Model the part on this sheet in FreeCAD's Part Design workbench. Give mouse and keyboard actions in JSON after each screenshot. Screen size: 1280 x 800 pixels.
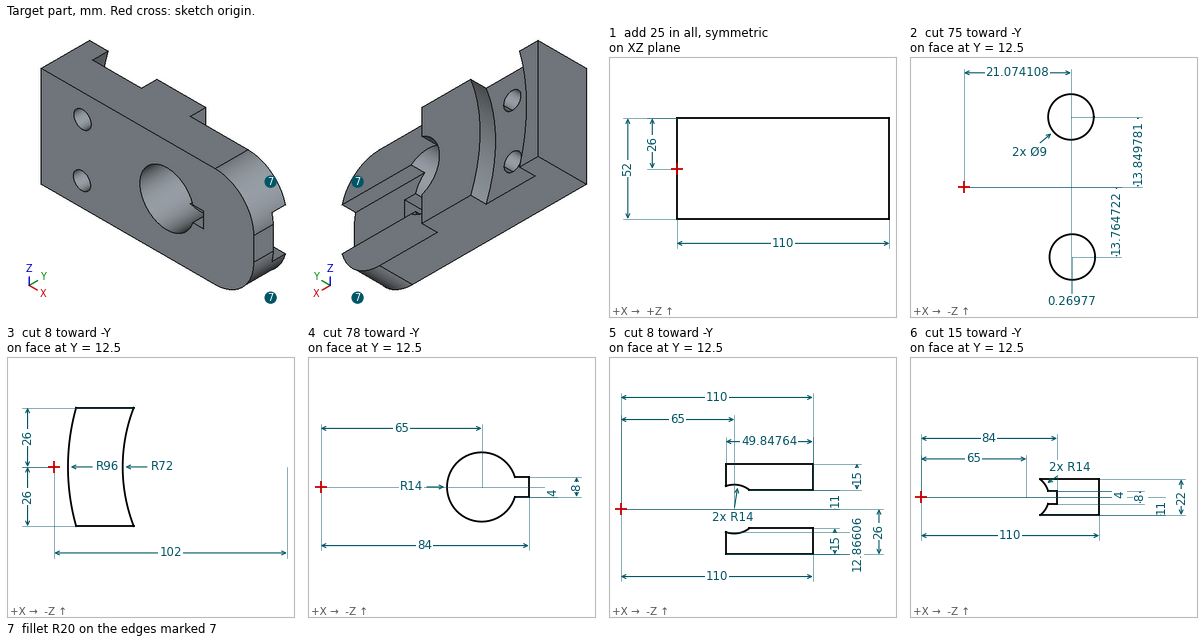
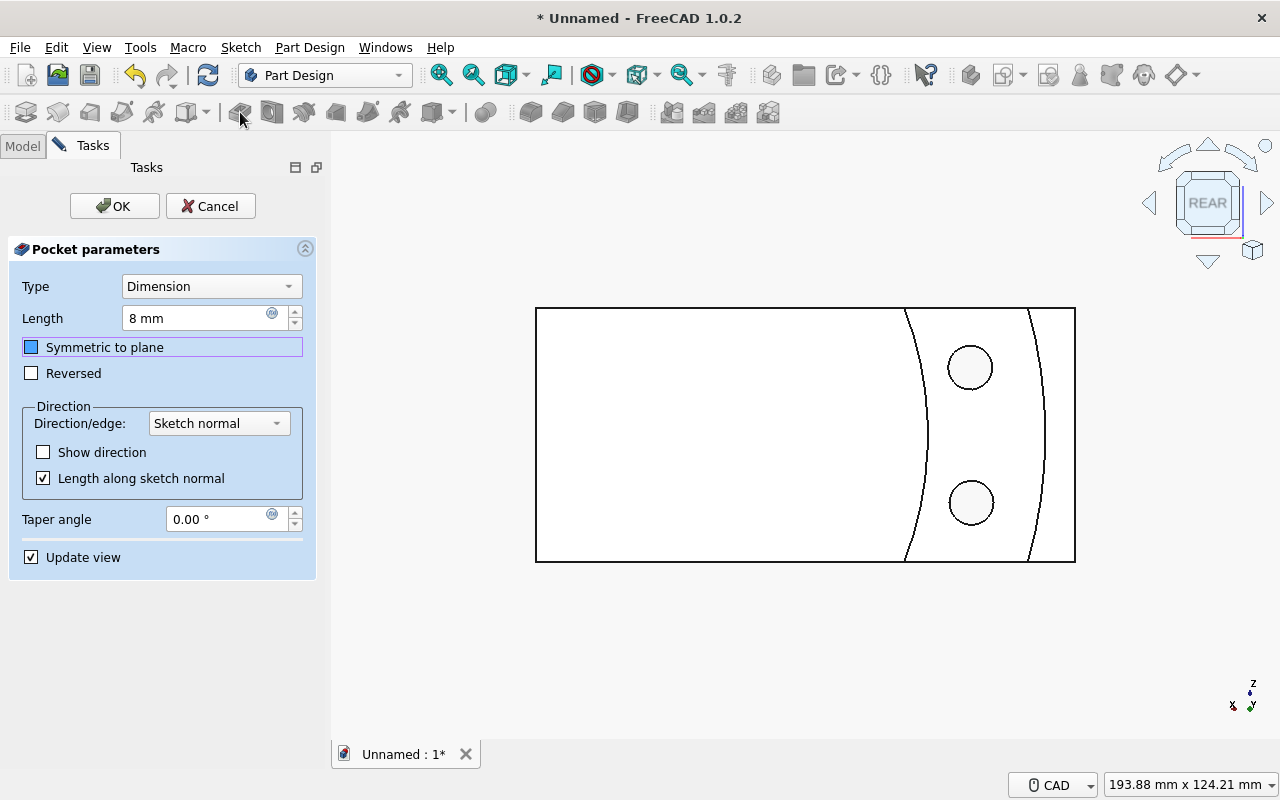
{"action": "left_click", "coordinate": [115, 206]}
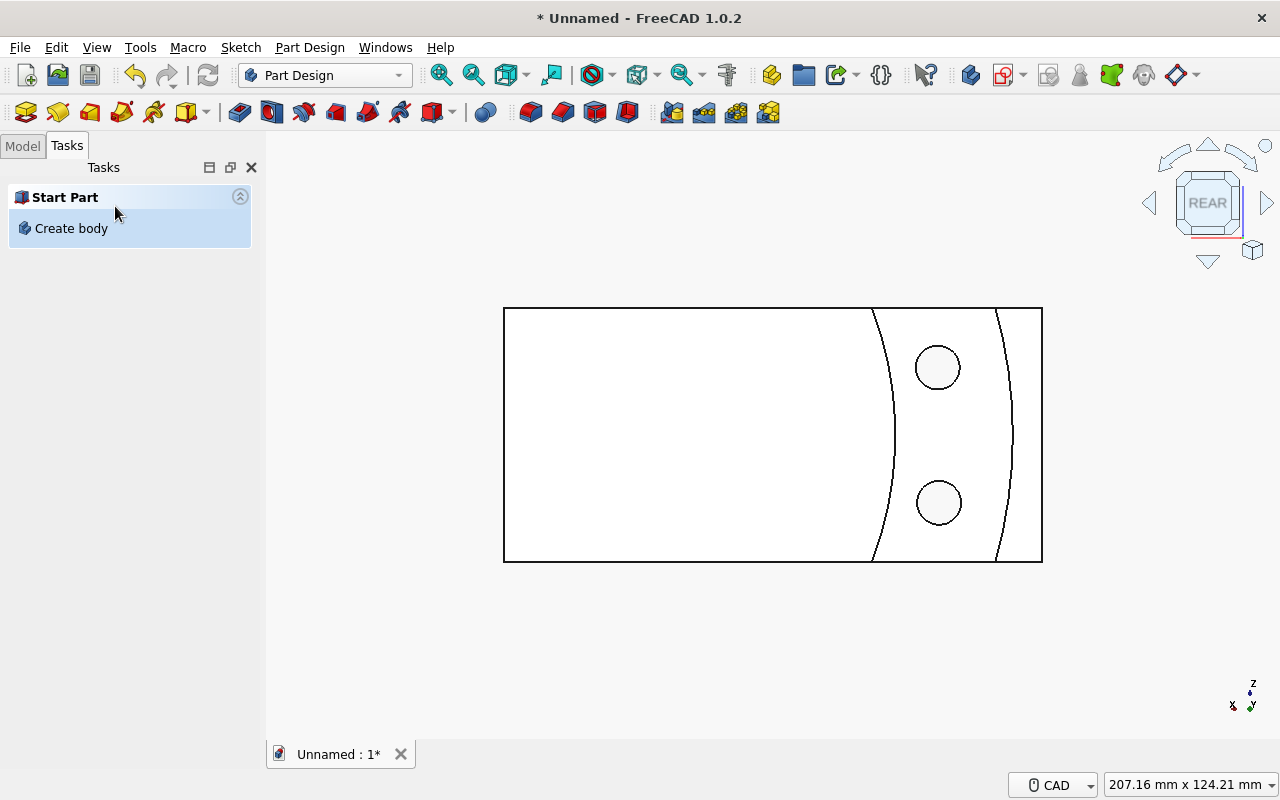
{"action": "left_click", "coordinate": [644, 434]}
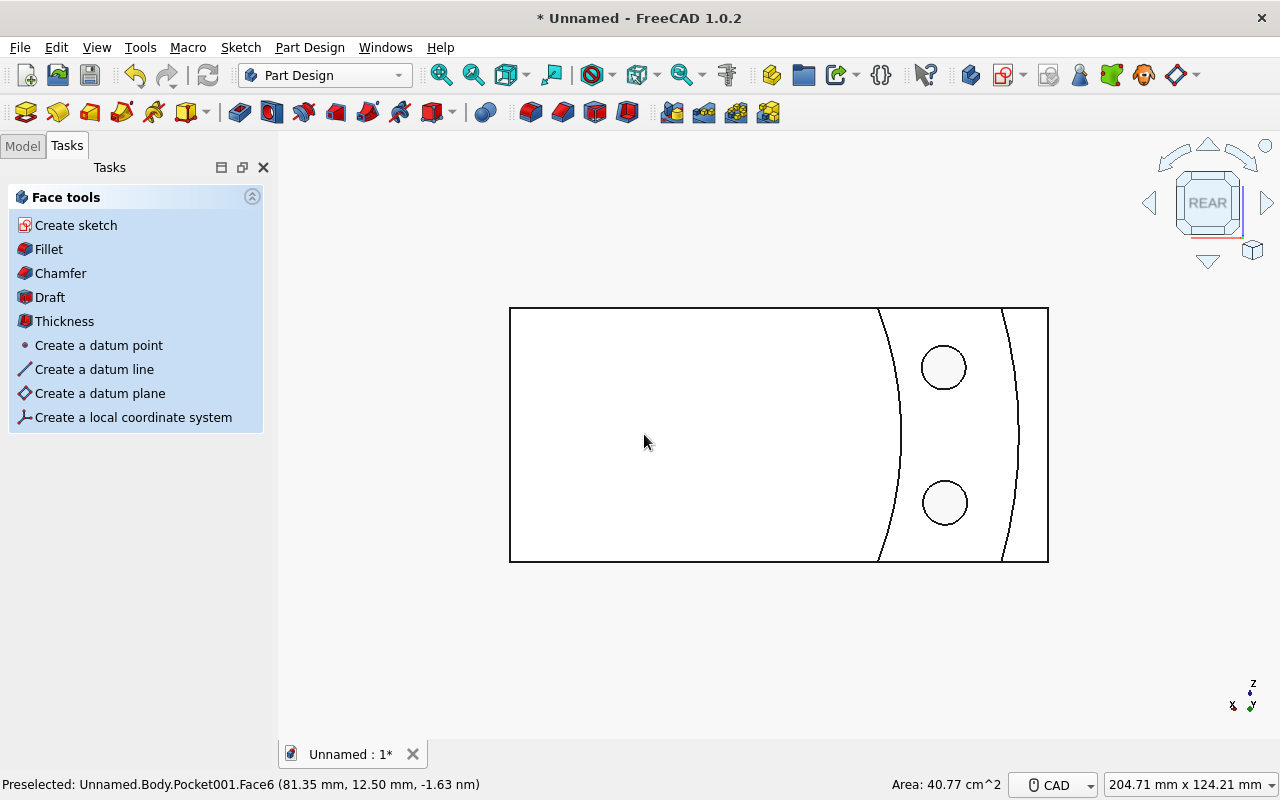
{"action": "left_click", "coordinate": [1004, 76]}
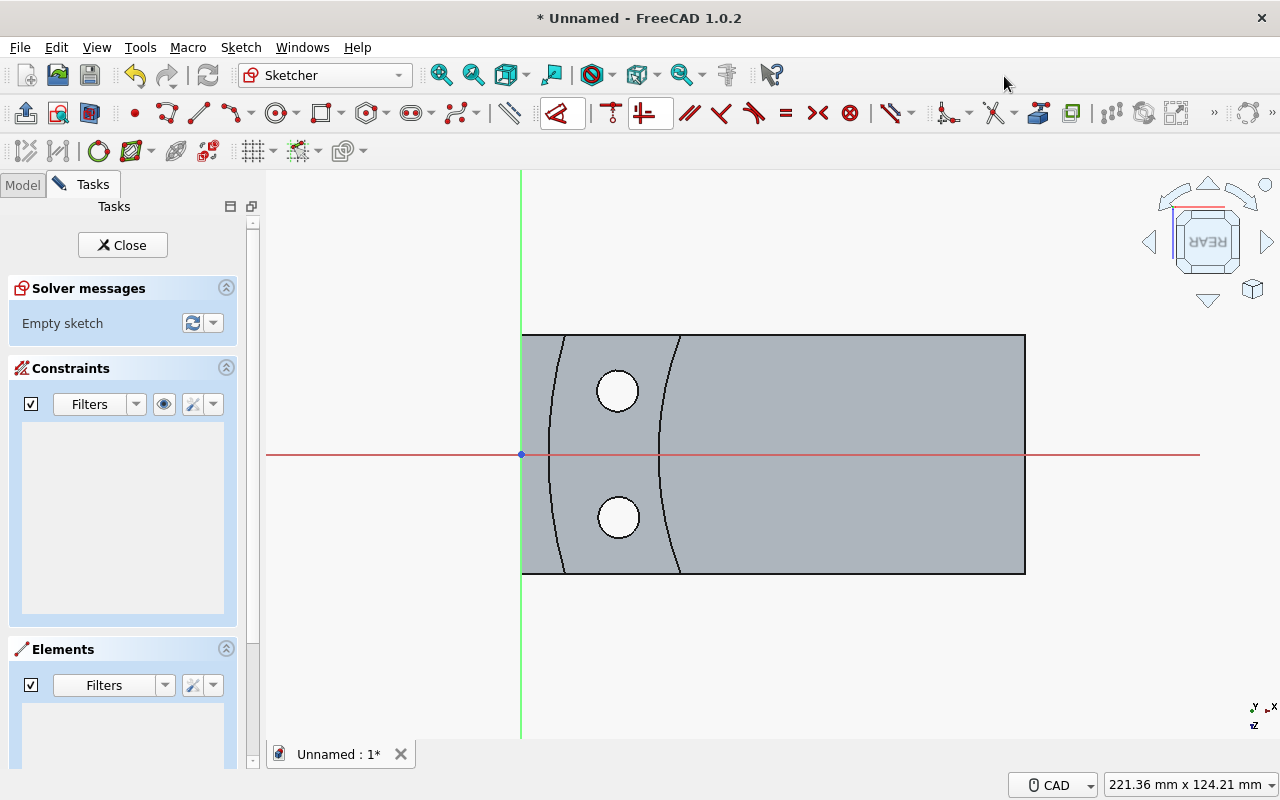
{"action": "scroll", "coordinate": [871, 454], "scroll_direction": "up", "scroll_amount": 7}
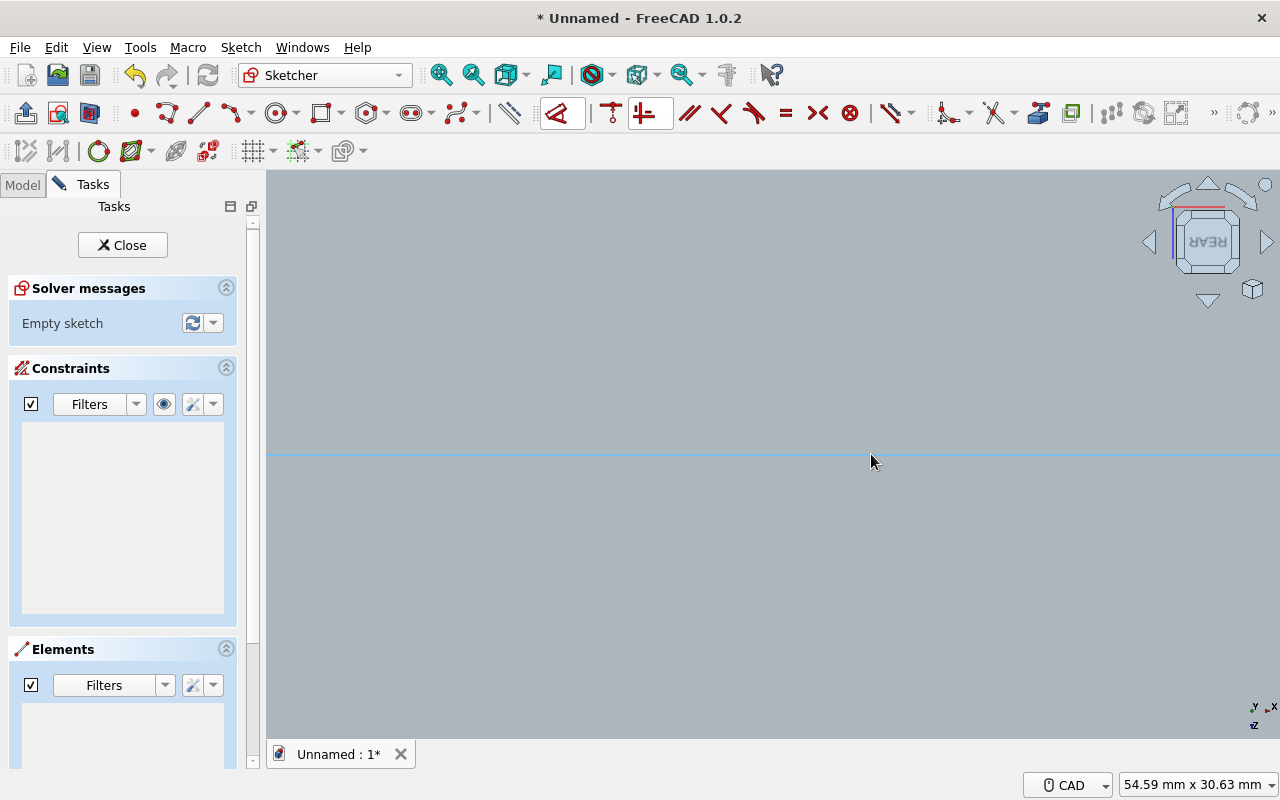
{"action": "left_click", "coordinate": [168, 114]}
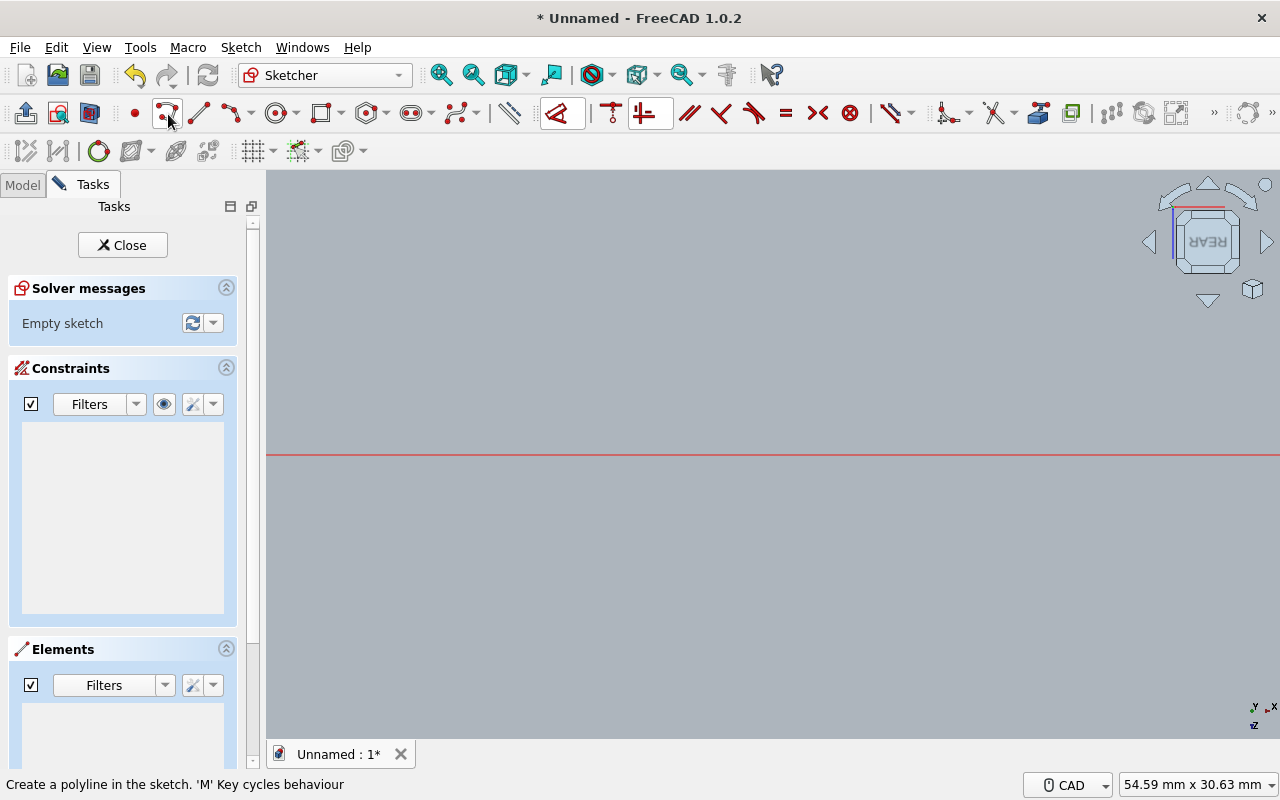
{"action": "left_click", "coordinate": [907, 529]}
{"action": "left_click", "coordinate": [1010, 529]}
{"action": "left_click", "coordinate": [1010, 380]}
{"action": "left_click", "coordinate": [907, 380]}
{"action": "right_click", "coordinate": [907, 380]}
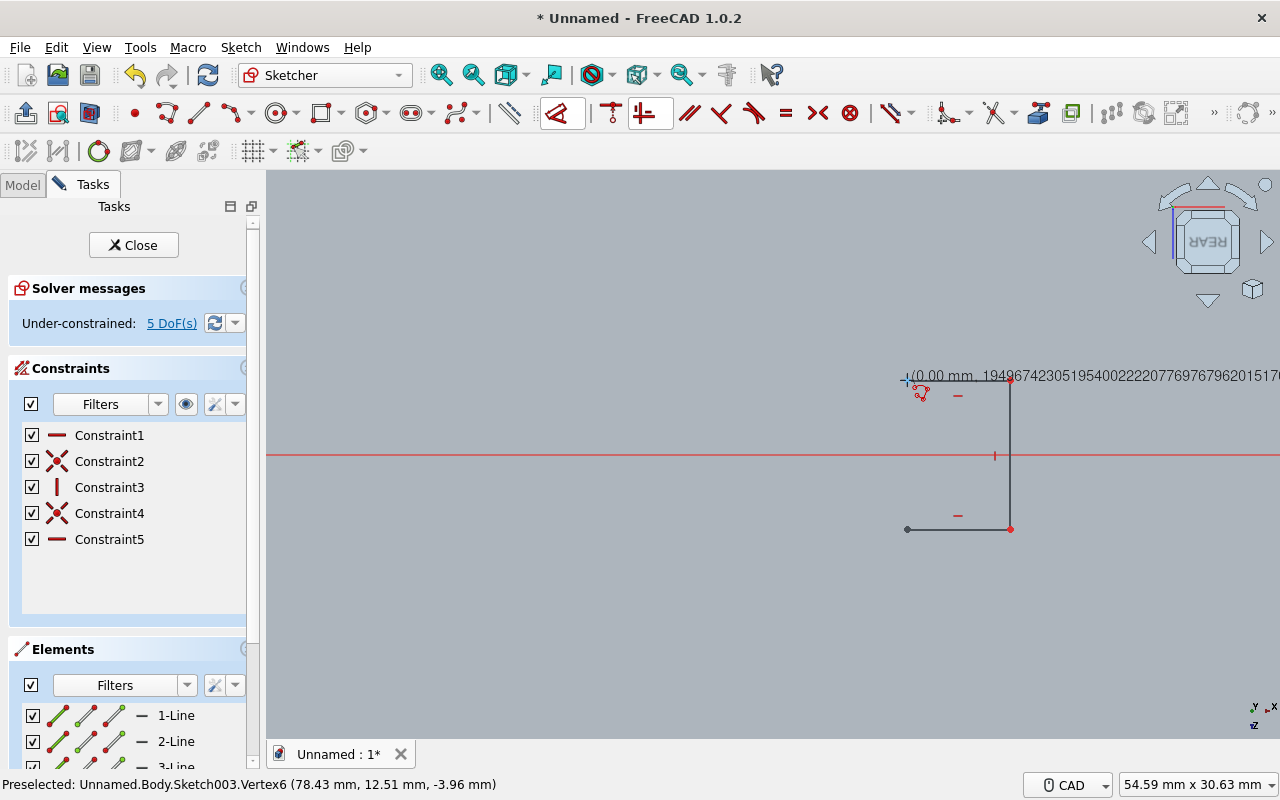
{"action": "left_click", "coordinate": [232, 114]}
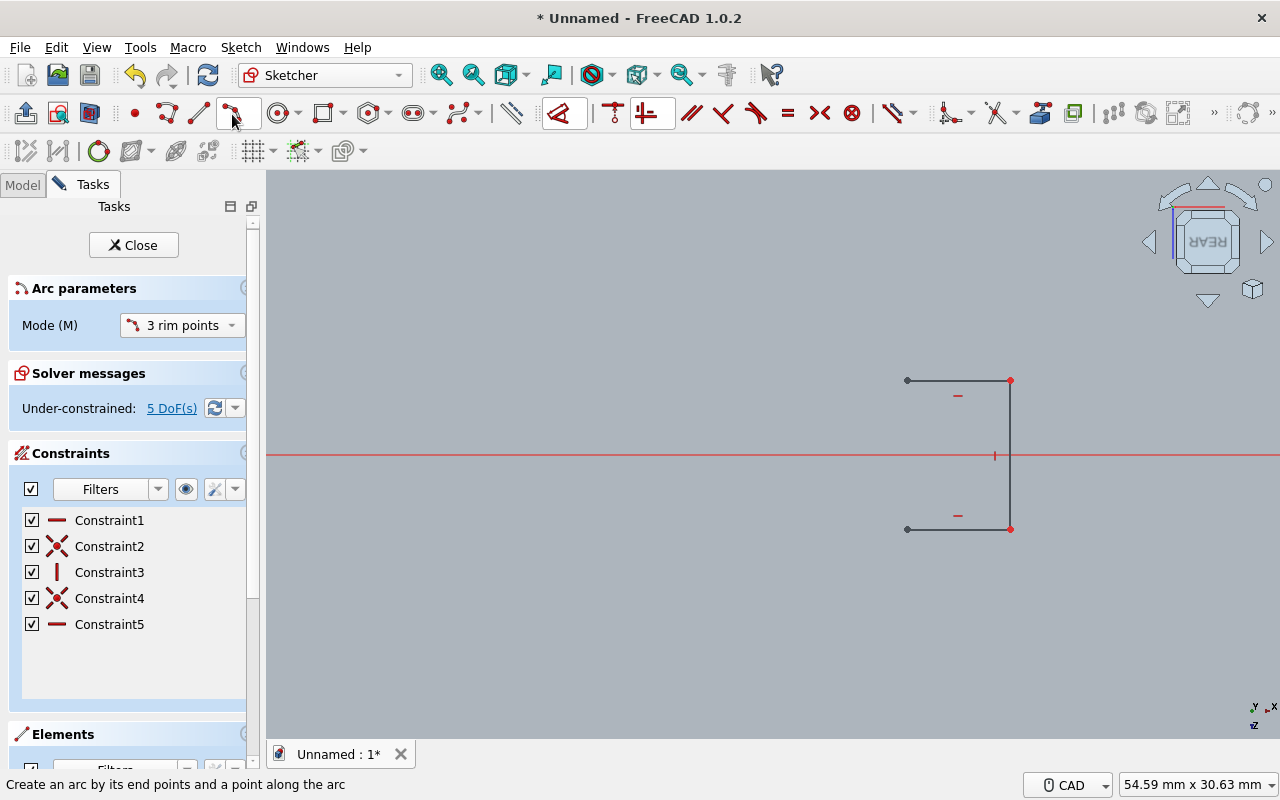
{"action": "left_click", "coordinate": [907, 381]}
{"action": "left_click", "coordinate": [907, 530]}
{"action": "left_click", "coordinate": [439, 314]}
{"action": "key", "text": "Escape"}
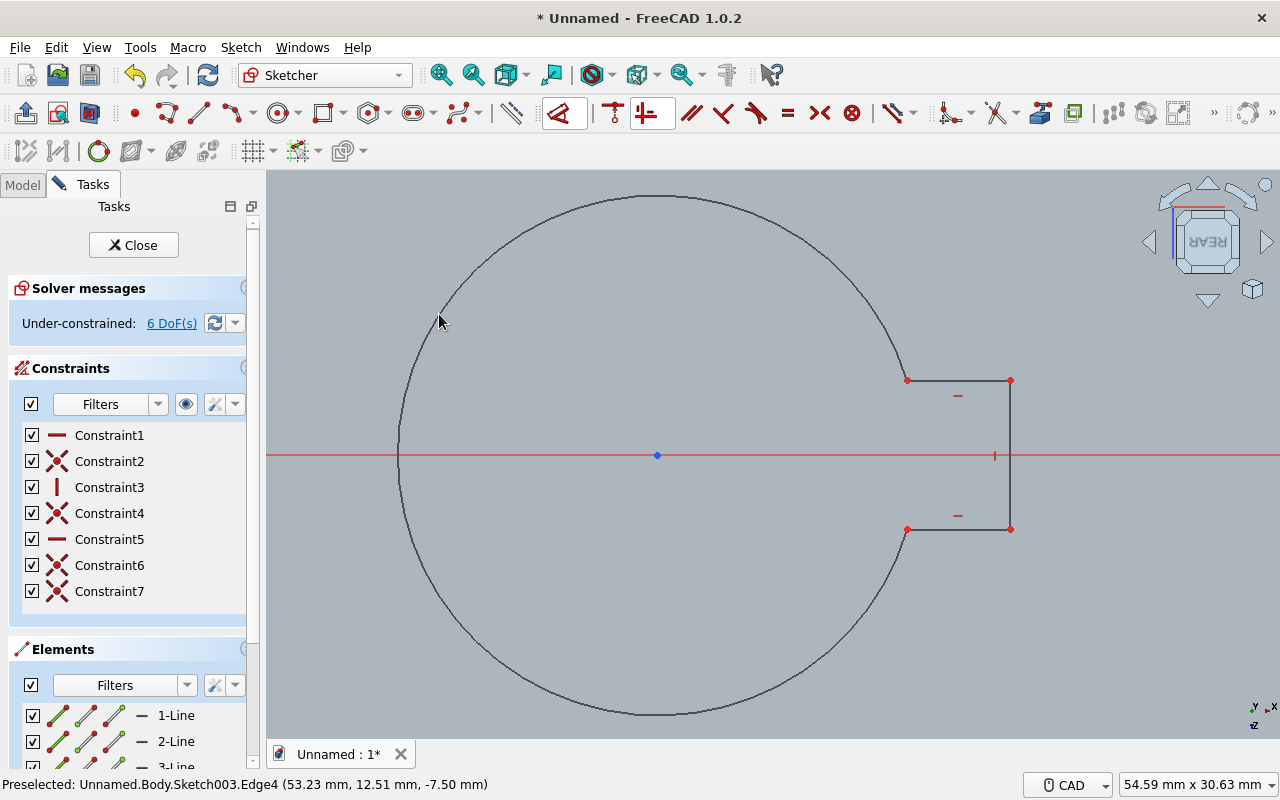
{"action": "left_click", "coordinate": [658, 456]}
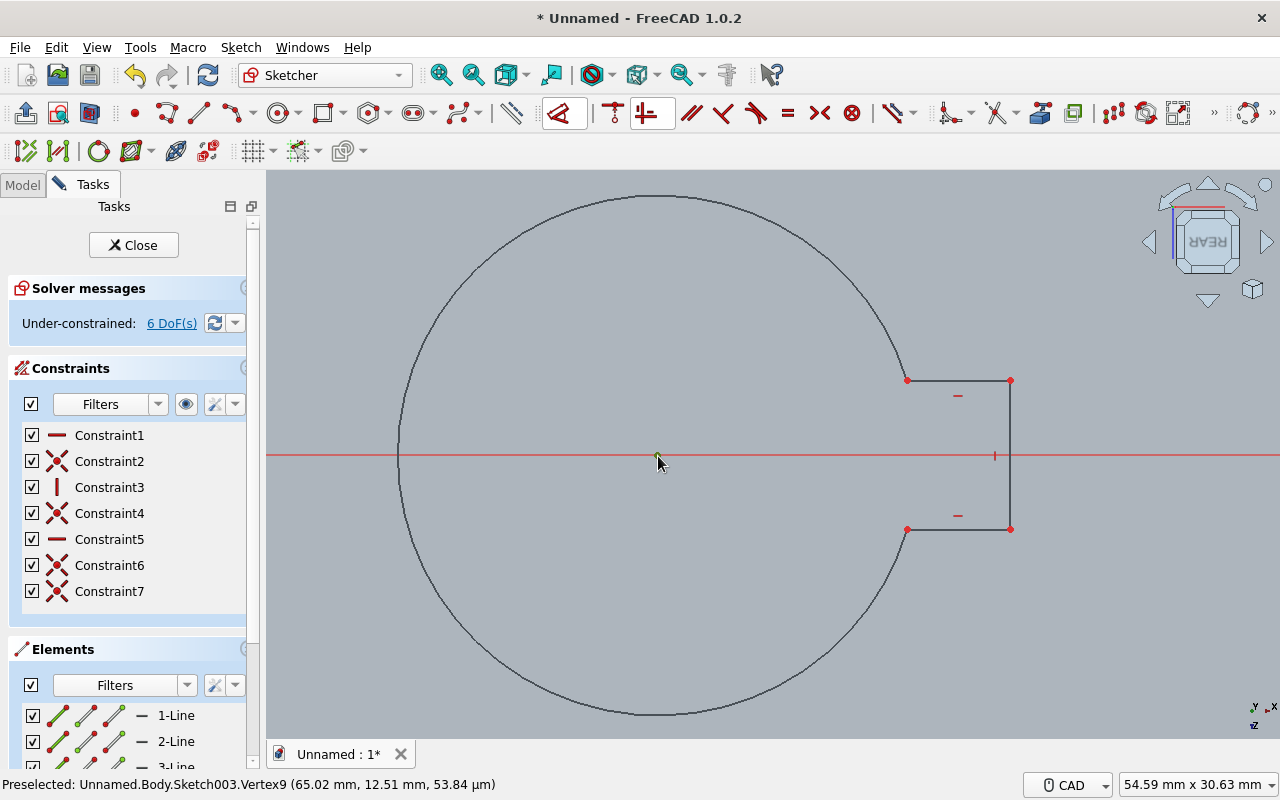
{"action": "left_click", "coordinate": [353, 454]}